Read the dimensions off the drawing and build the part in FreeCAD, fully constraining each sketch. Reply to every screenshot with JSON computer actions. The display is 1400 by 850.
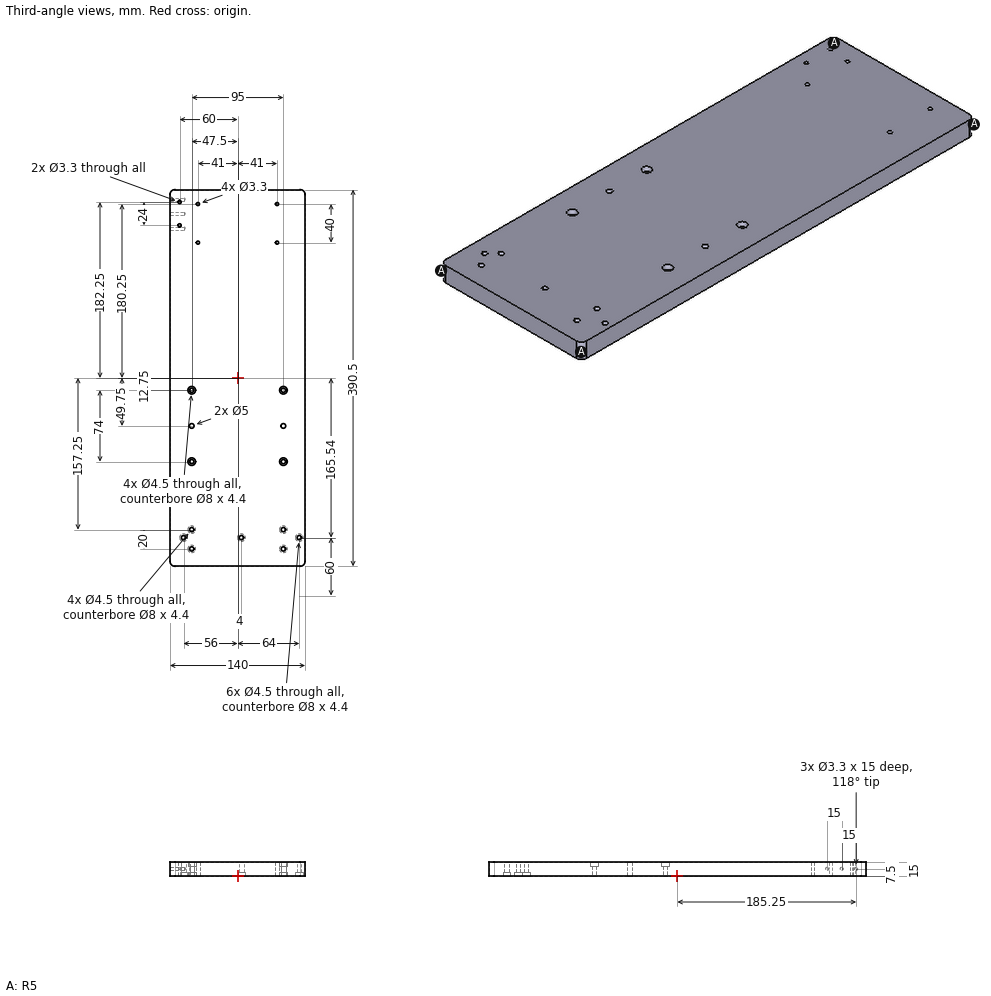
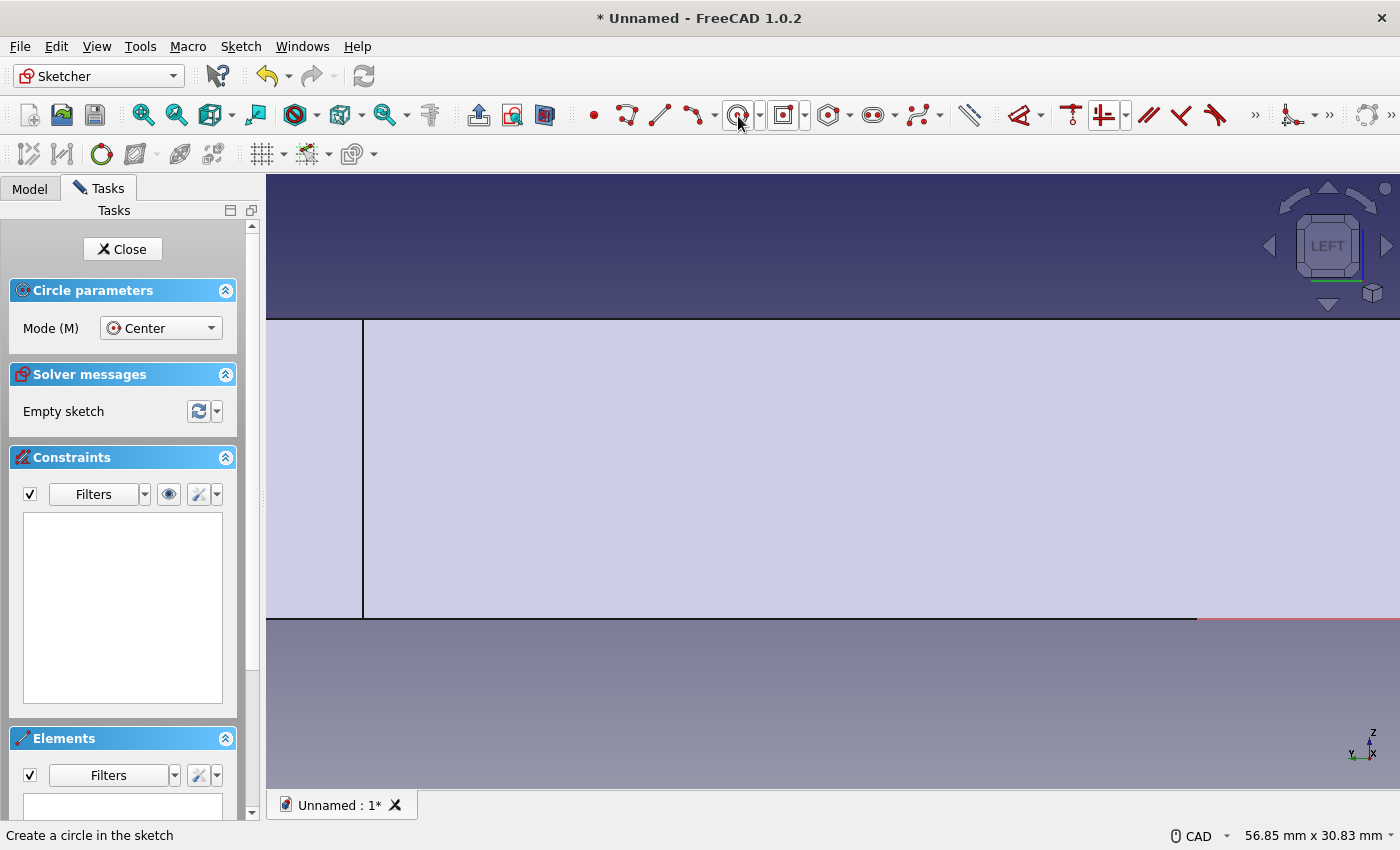
{"action": "left_click", "coordinate": [462, 469]}
{"action": "mouse_move", "coordinate": [486, 446]}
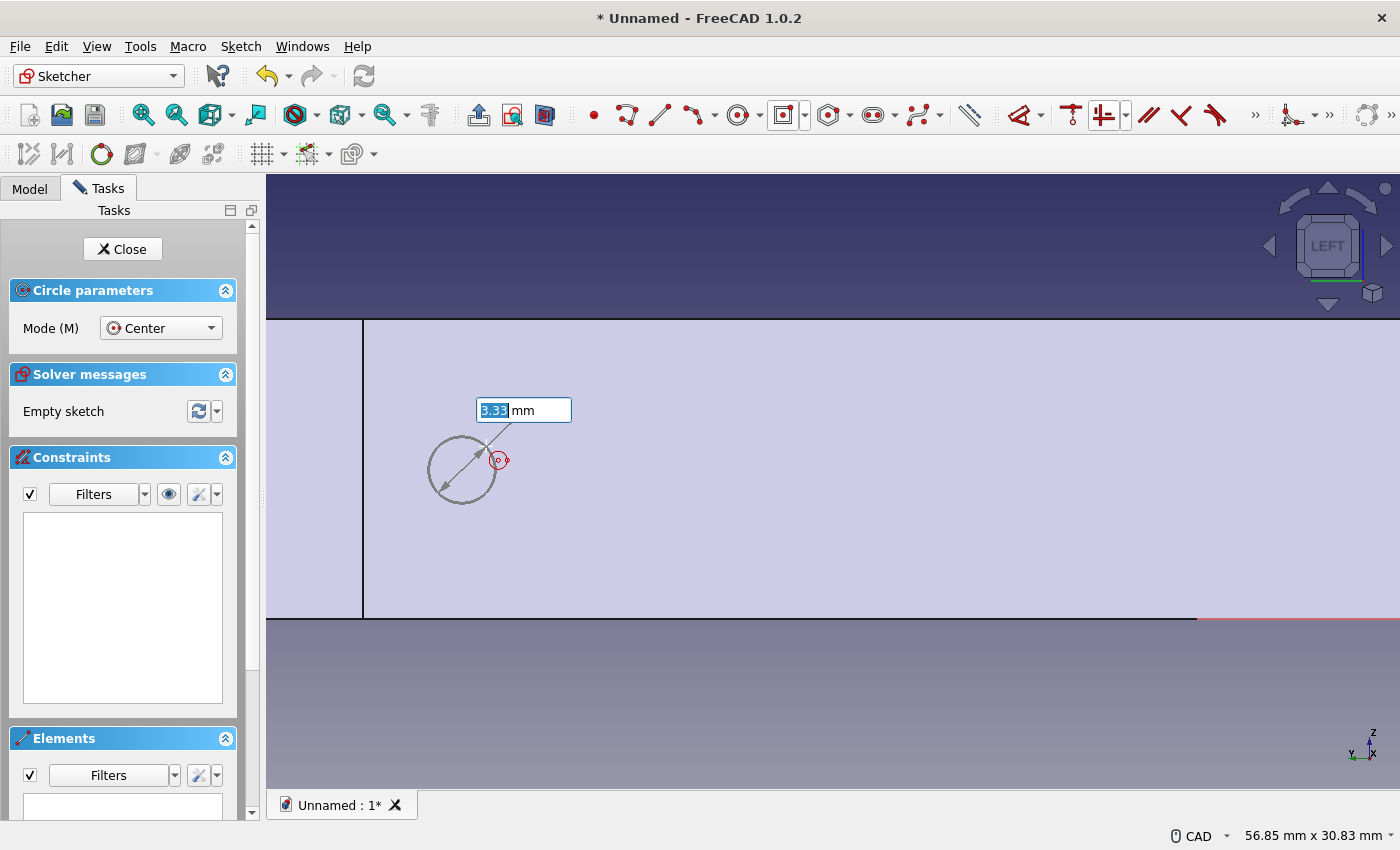
{"action": "type", "text": "3.3"}
{"action": "key", "text": "Return"}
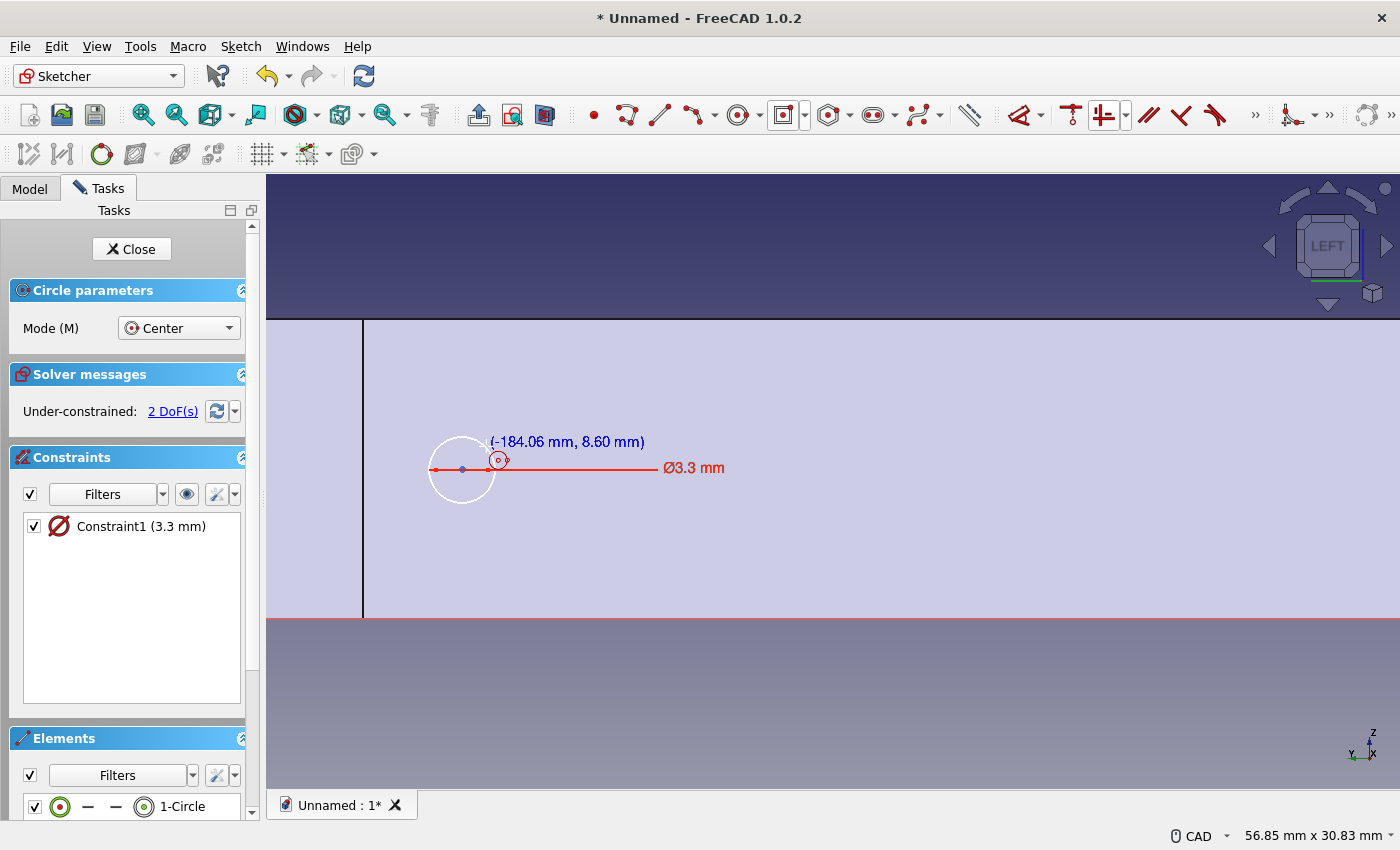
{"action": "left_click", "coordinate": [762, 469]}
{"action": "mouse_move", "coordinate": [785, 446]}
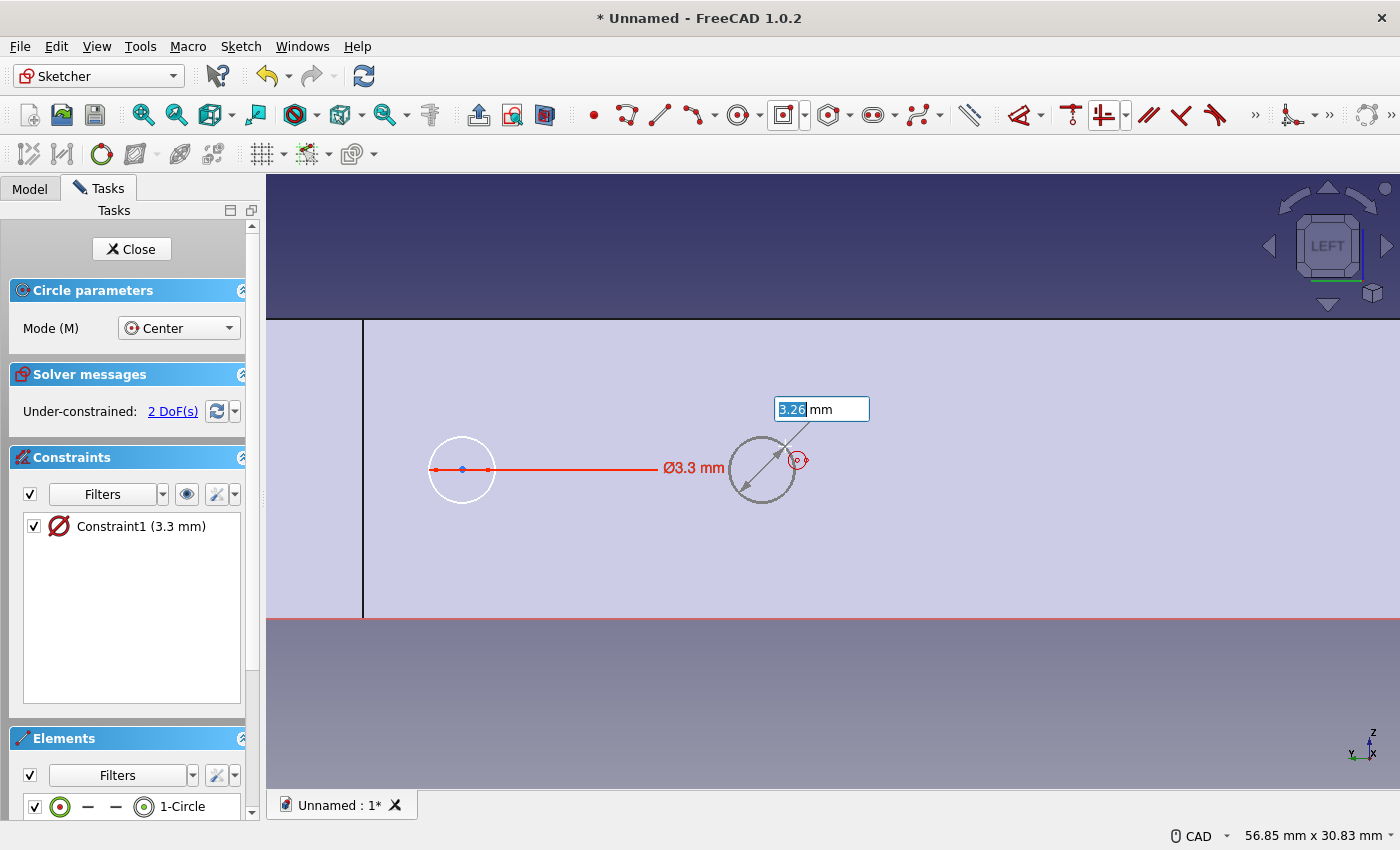
{"action": "type", "text": "3.3"}
{"action": "key", "text": "Return"}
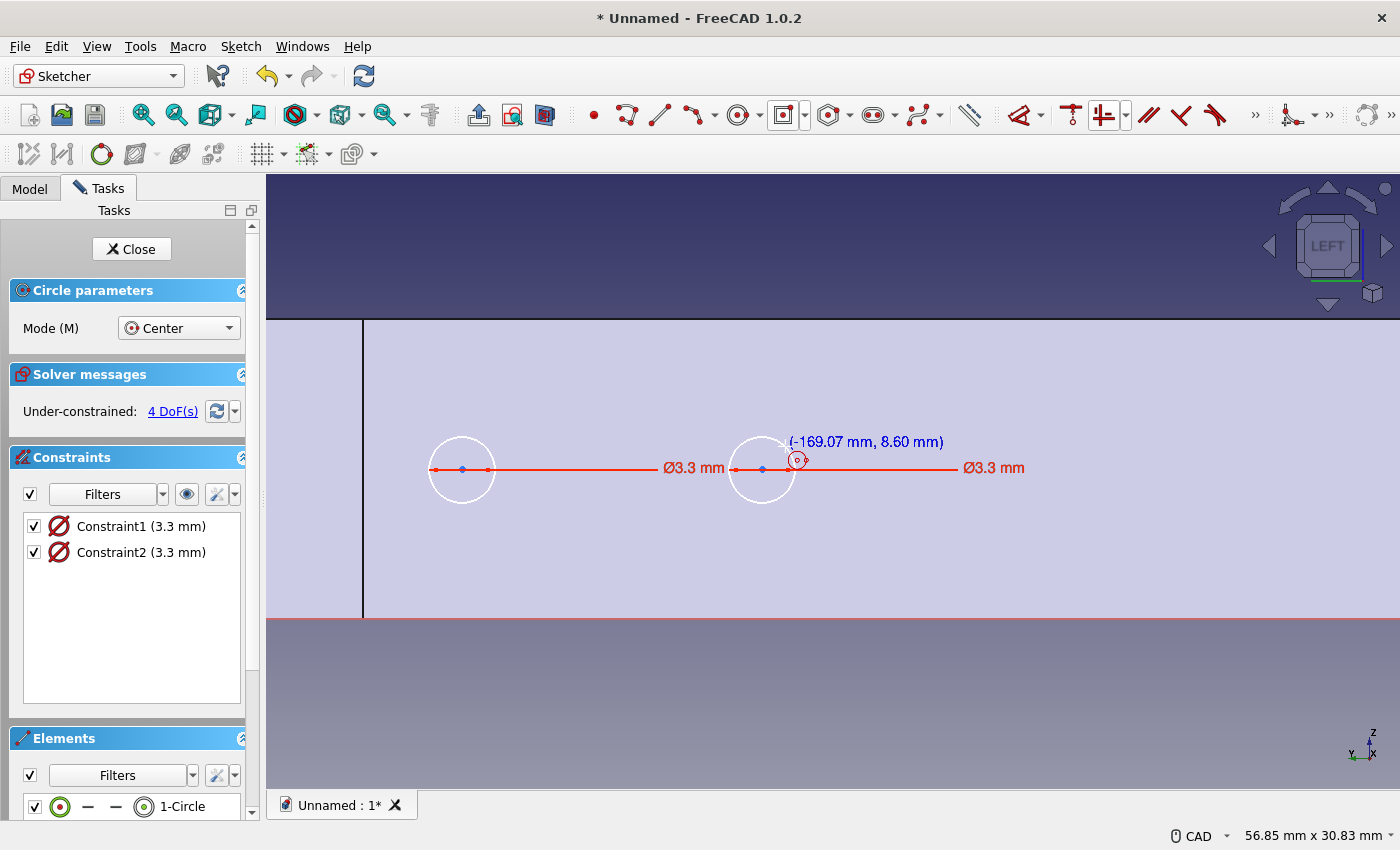
{"action": "left_click", "coordinate": [1061, 469]}
{"action": "mouse_move", "coordinate": [1084, 446]}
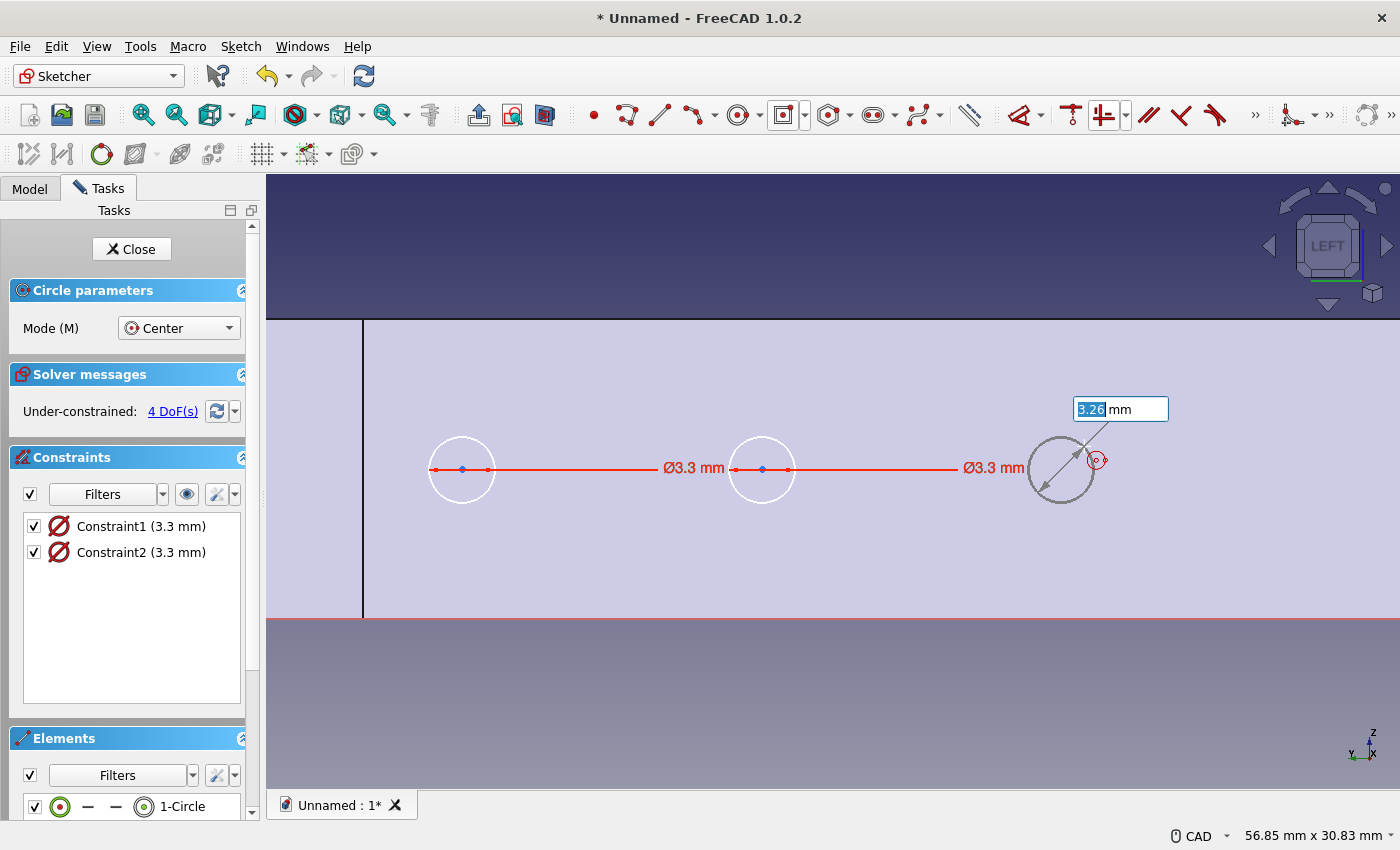
{"action": "type", "text": "3.3"}
{"action": "key", "text": "Return"}
{"action": "key", "text": "Escape"}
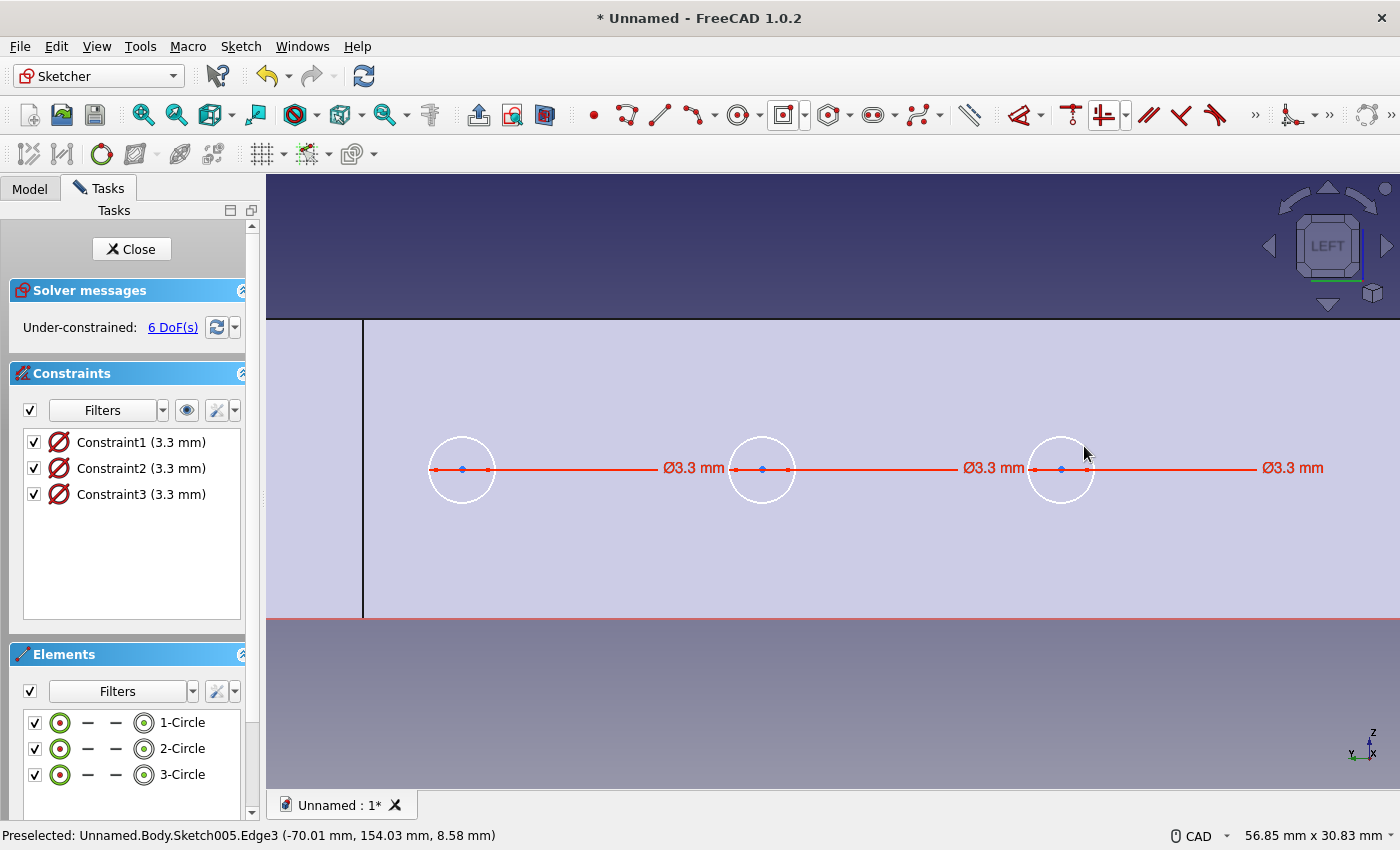
{"action": "left_click", "coordinate": [462, 470]}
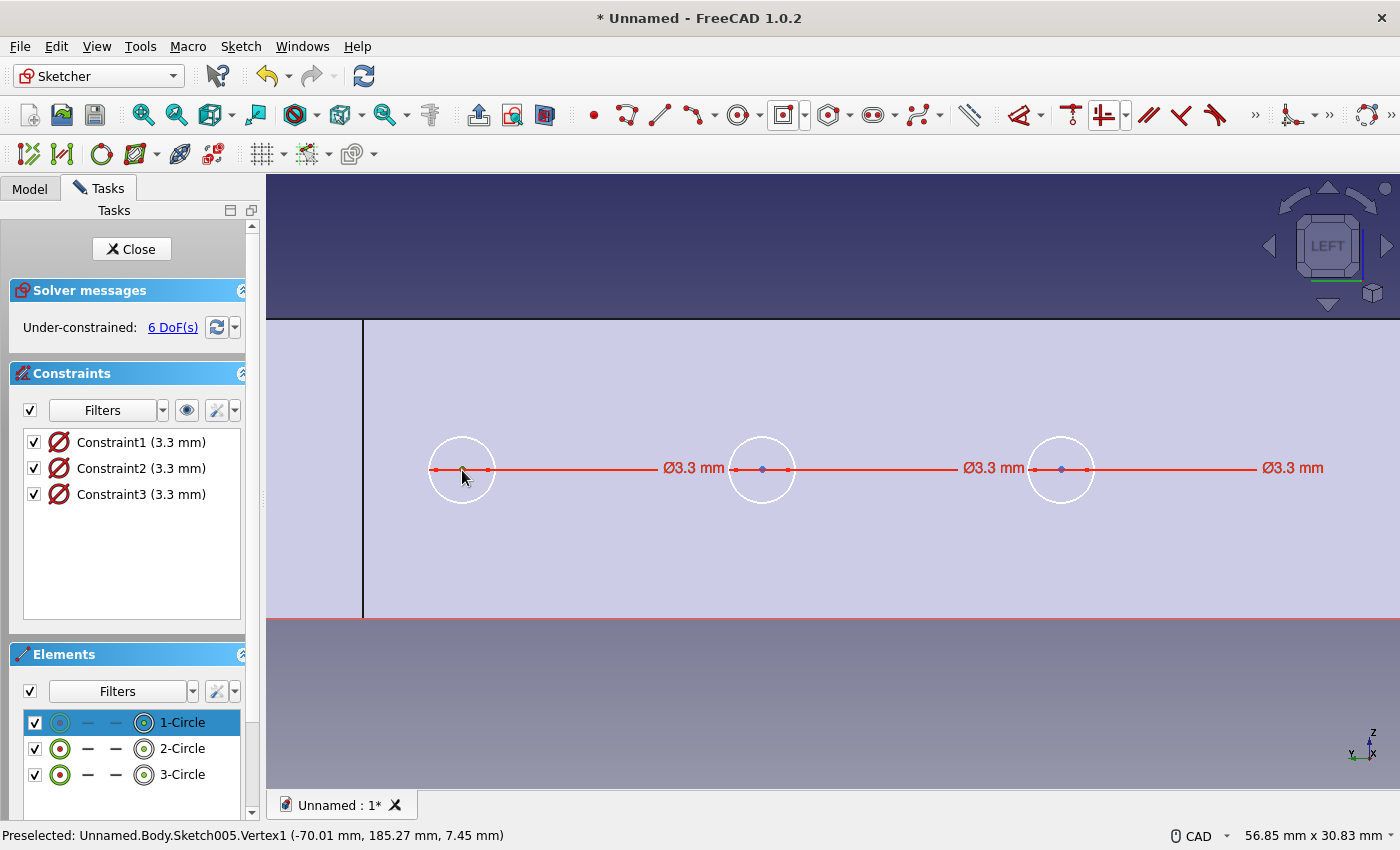
{"action": "left_click", "coordinate": [762, 470]}